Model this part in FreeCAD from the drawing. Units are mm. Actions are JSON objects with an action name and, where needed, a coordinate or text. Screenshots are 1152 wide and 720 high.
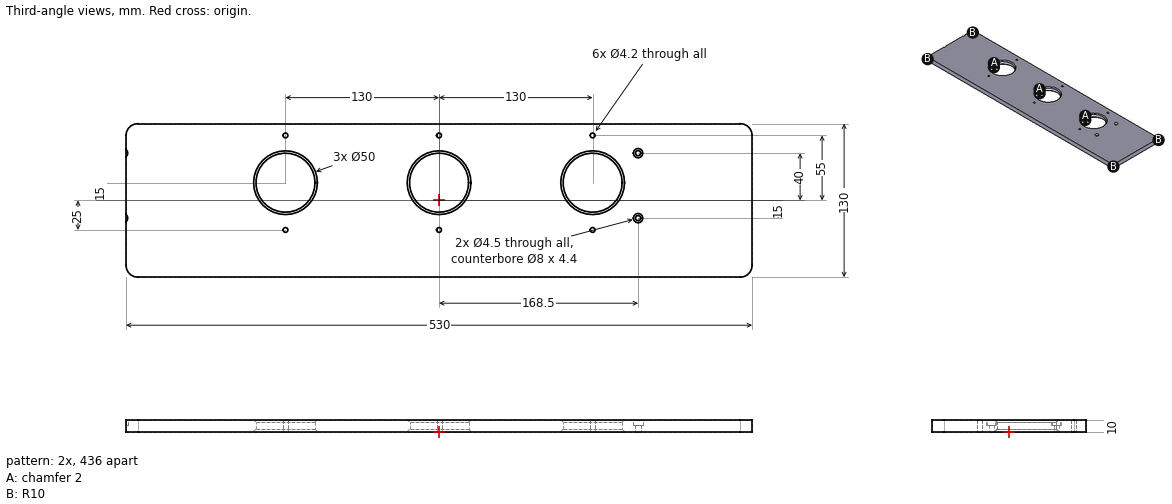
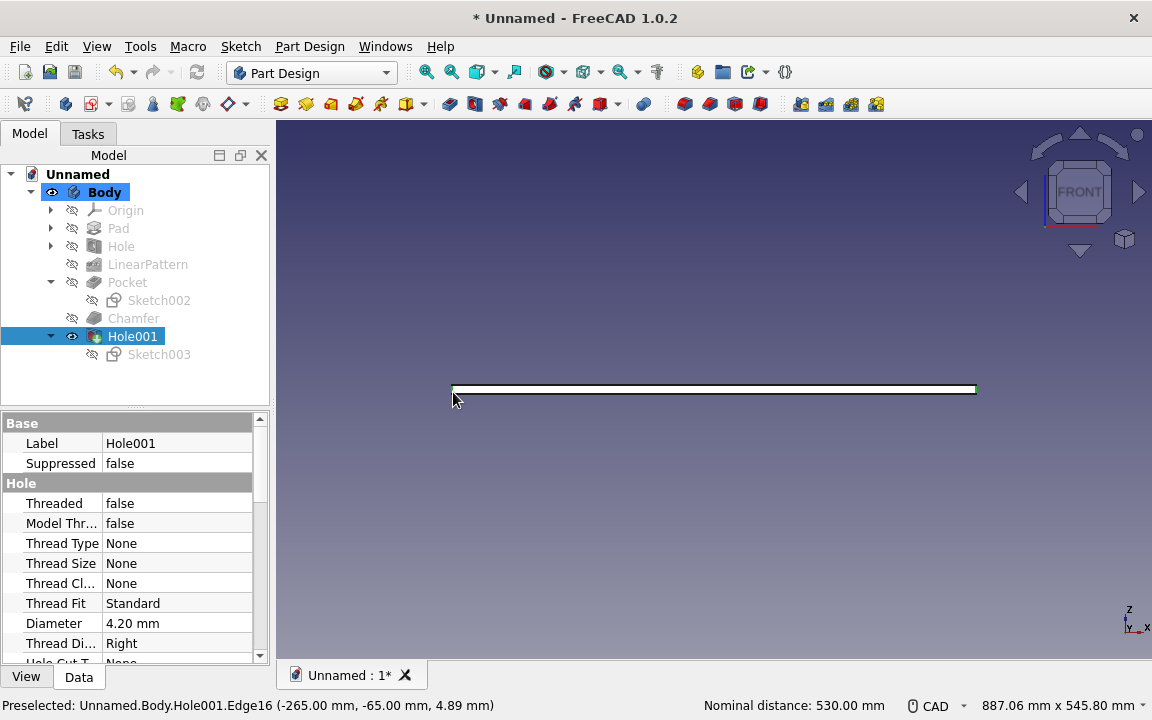
{"action": "key", "text": "3"}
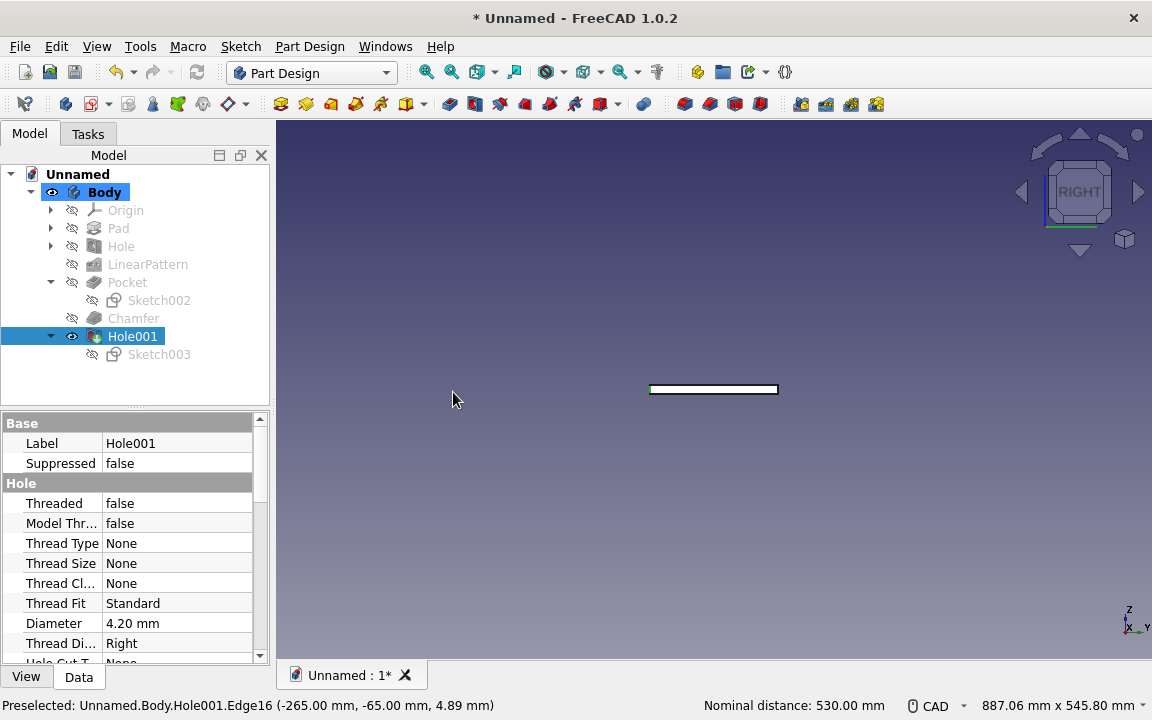
{"action": "left_click", "coordinate": [427, 72]}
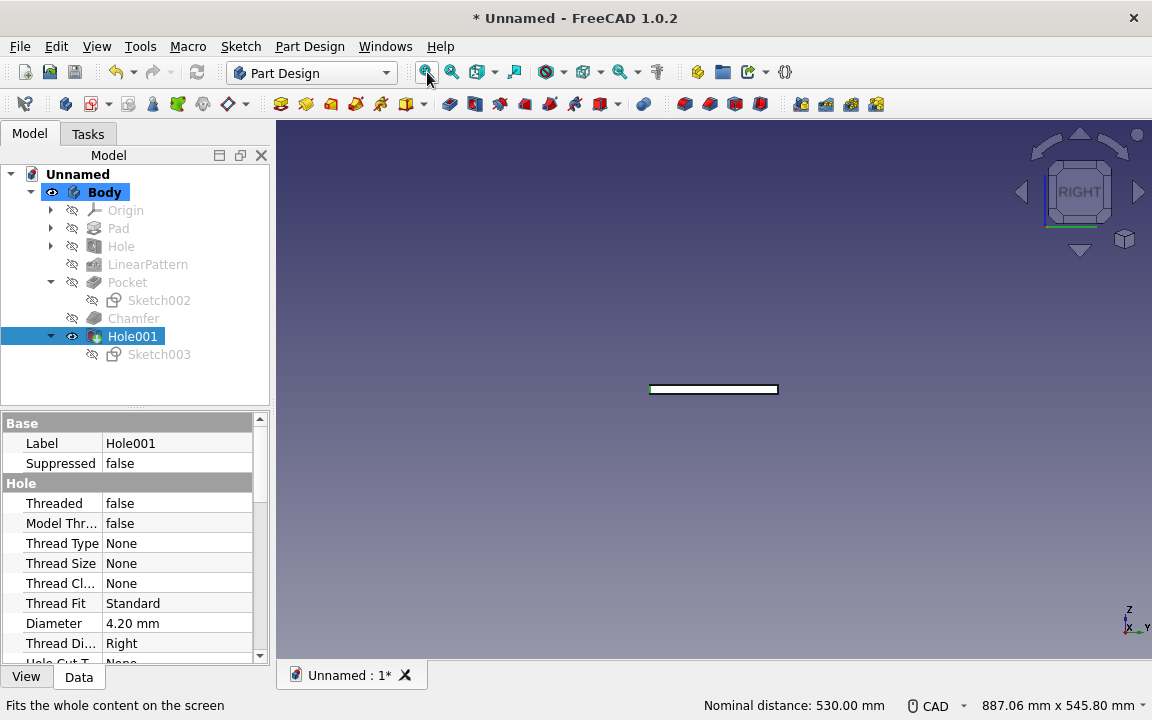
{"action": "scroll", "coordinate": [778, 388], "scroll_direction": "up", "scroll_amount": 7}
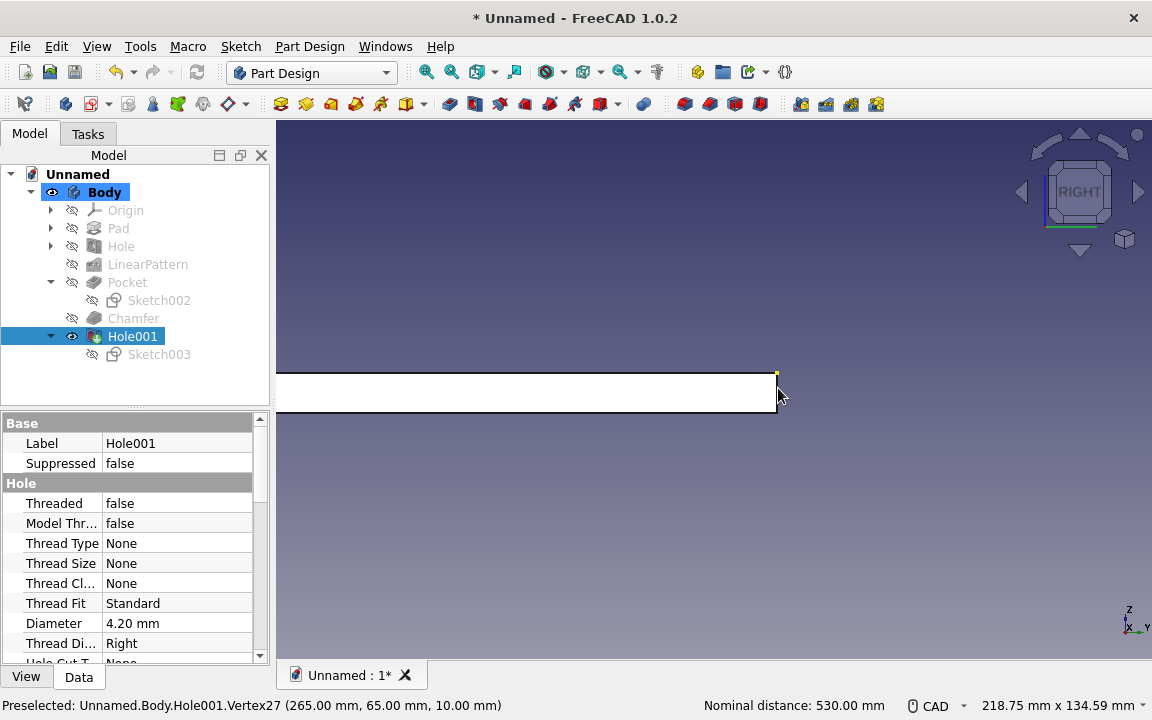
{"action": "left_click", "coordinate": [777, 392], "text": "ctrl"}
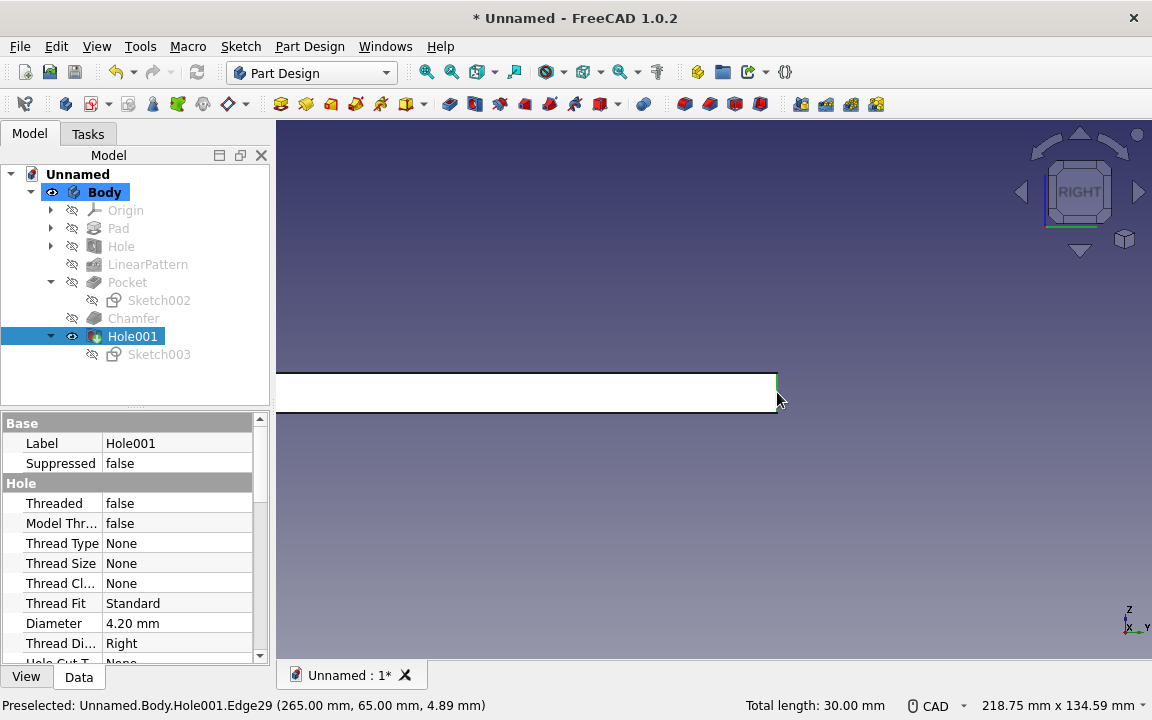
{"action": "left_click", "coordinate": [427, 72]}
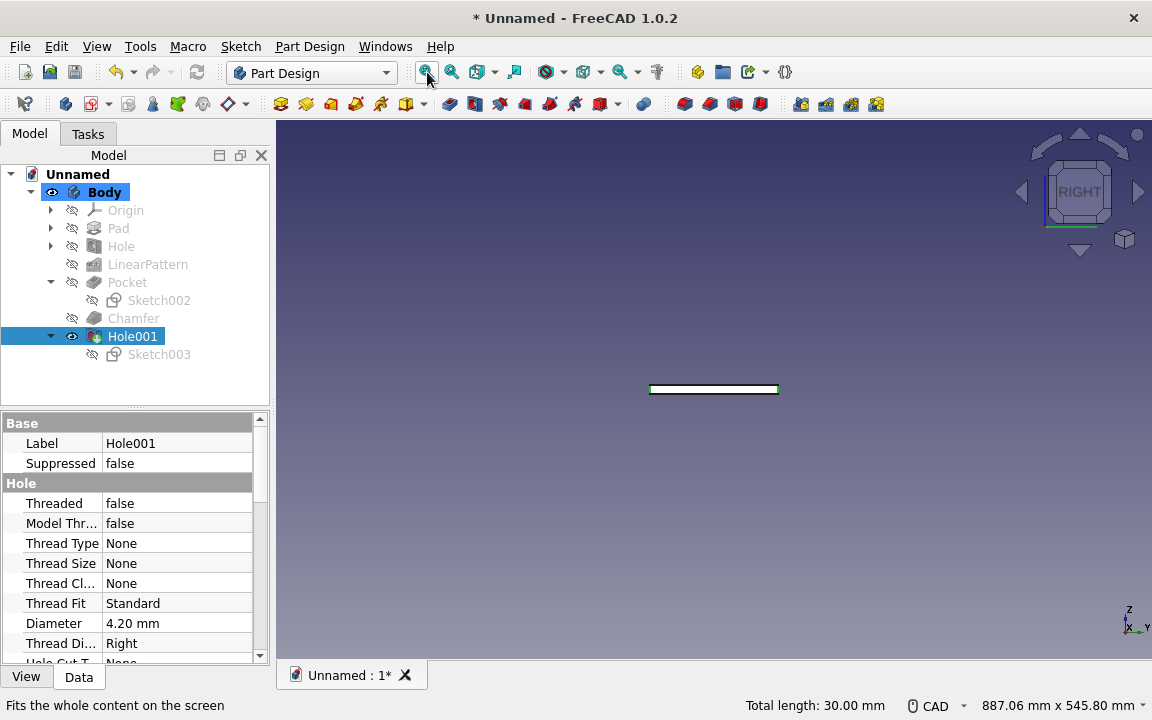
{"action": "key", "text": "5"}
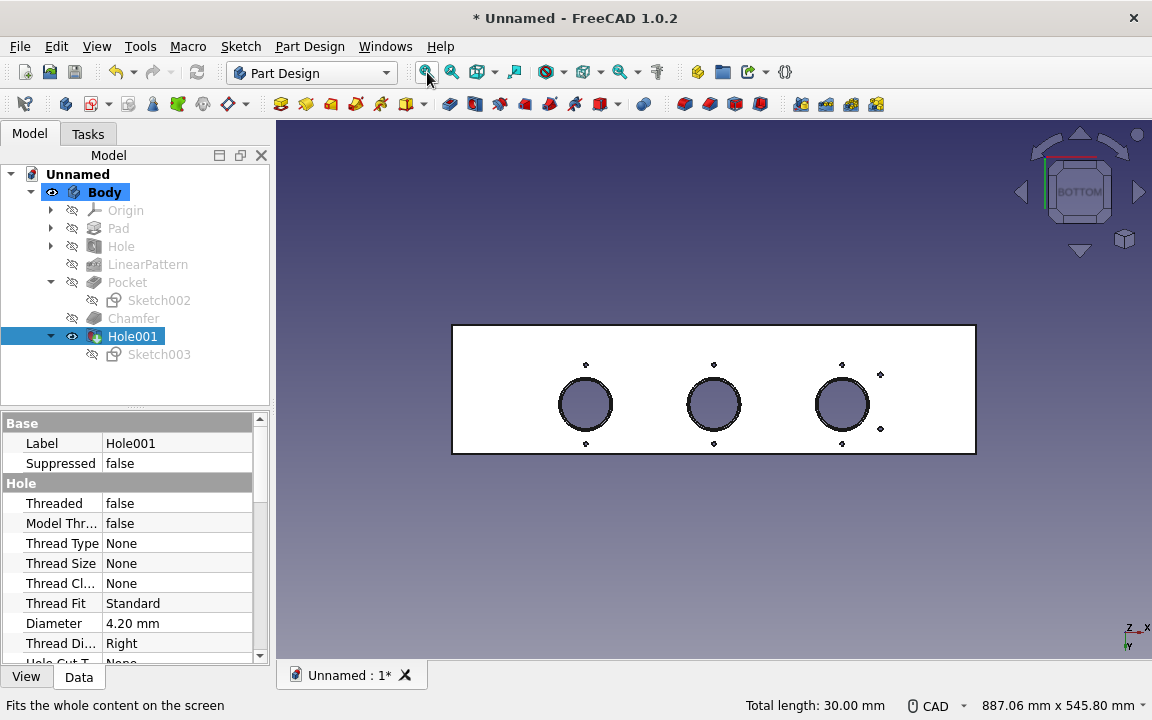
{"action": "scroll", "coordinate": [452, 453], "scroll_direction": "up", "scroll_amount": 7}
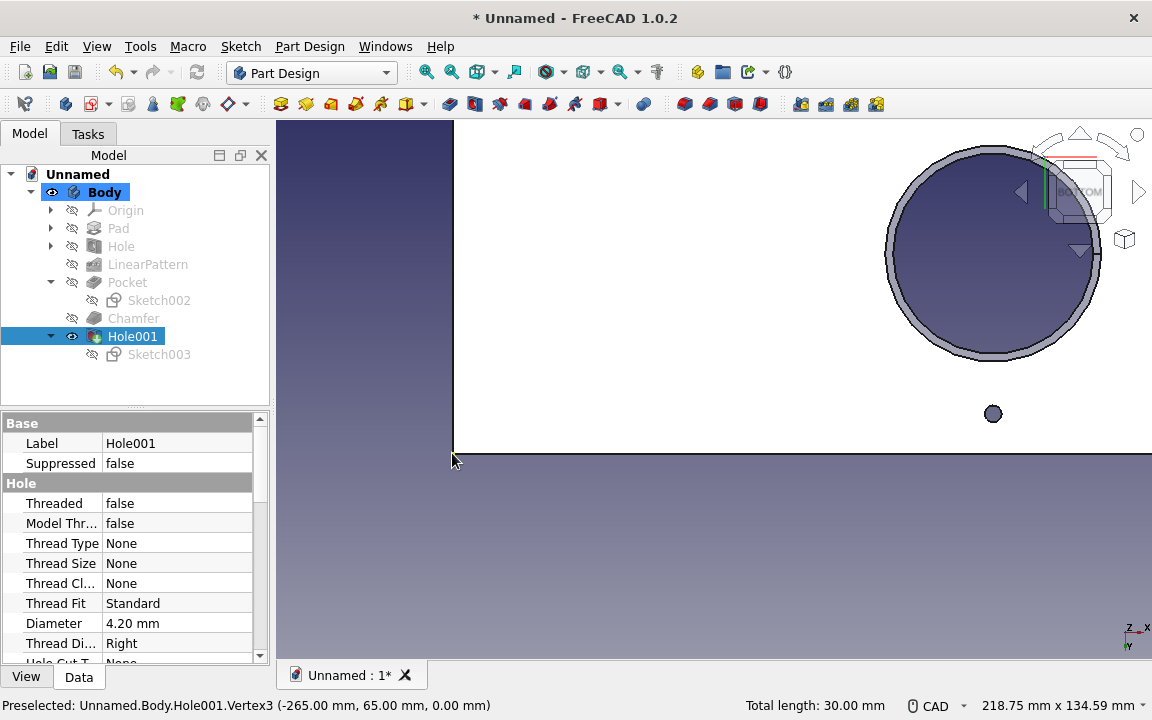
{"action": "left_click", "coordinate": [427, 72]}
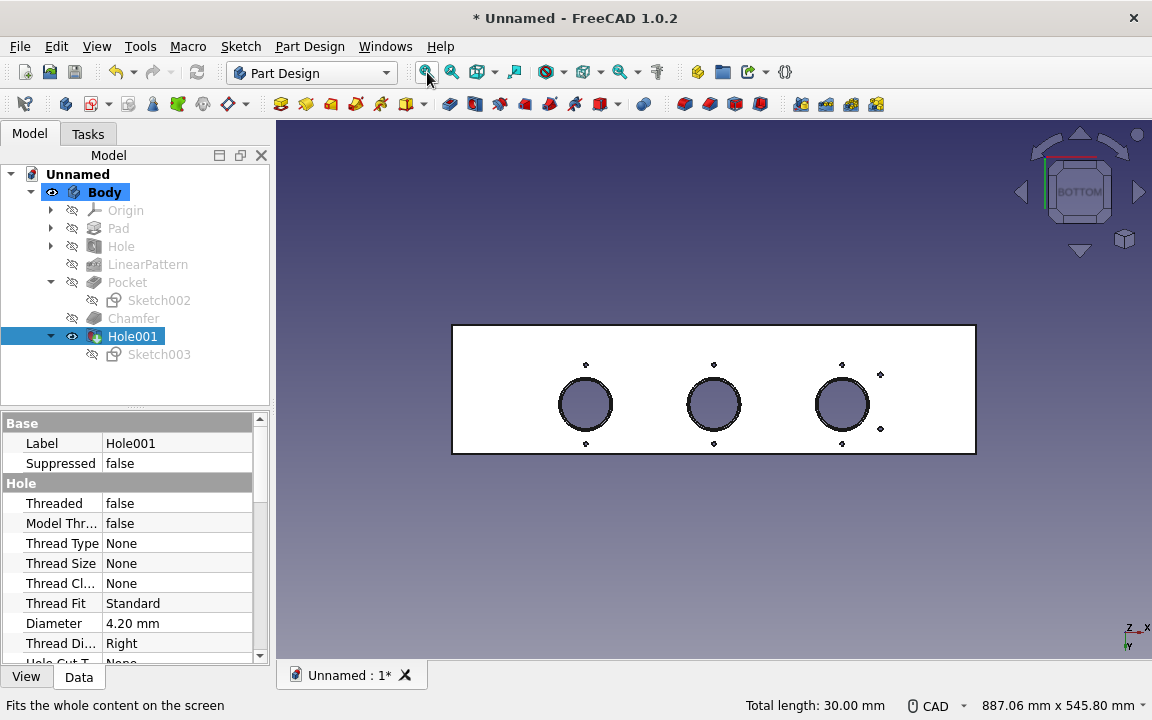
{"action": "key", "text": "4"}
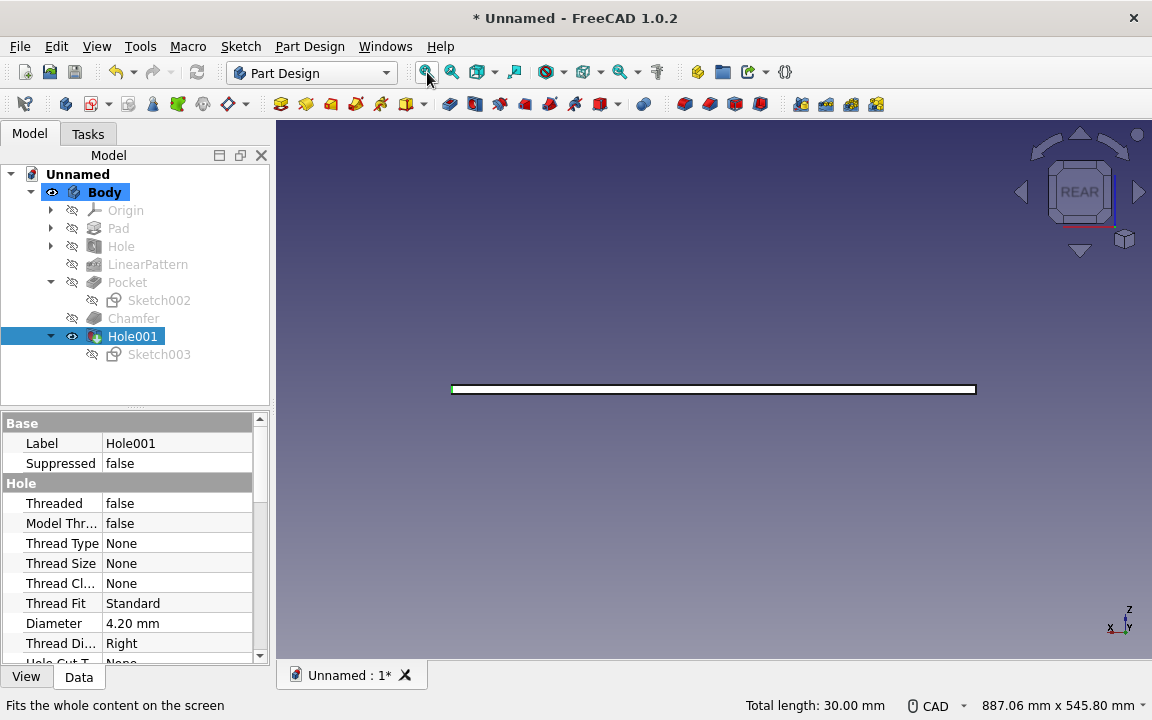
{"action": "scroll", "coordinate": [976, 388], "scroll_direction": "up", "scroll_amount": 7}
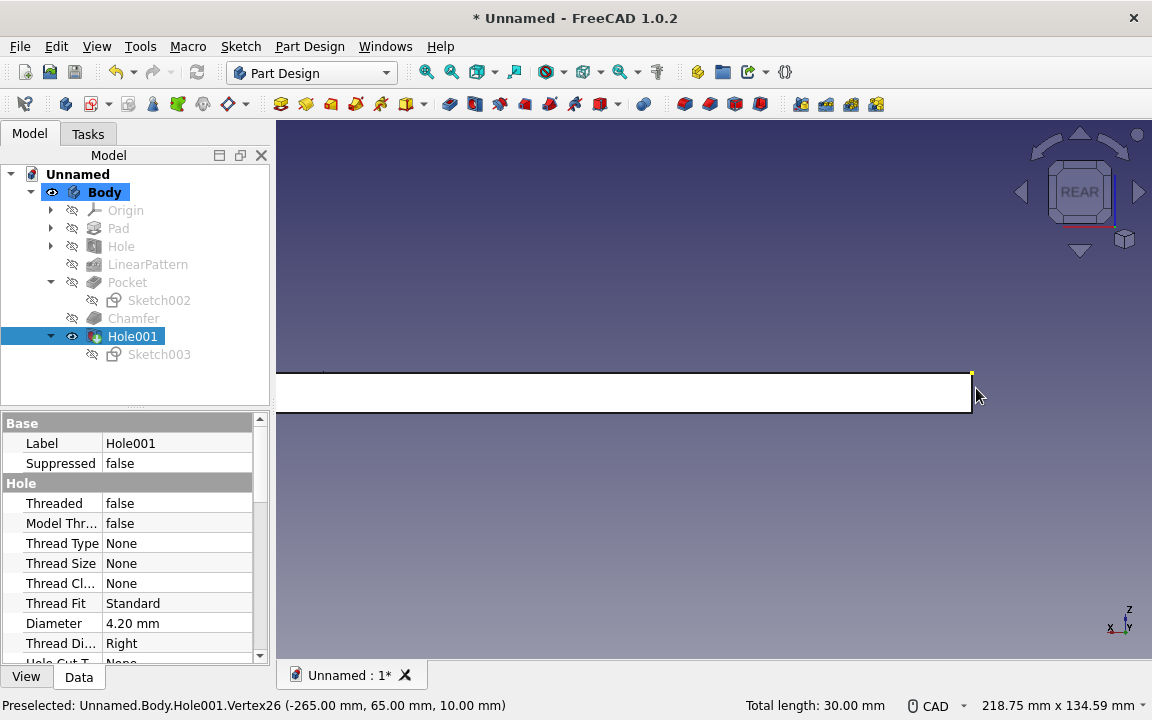
{"action": "left_click", "coordinate": [972, 392], "text": "ctrl"}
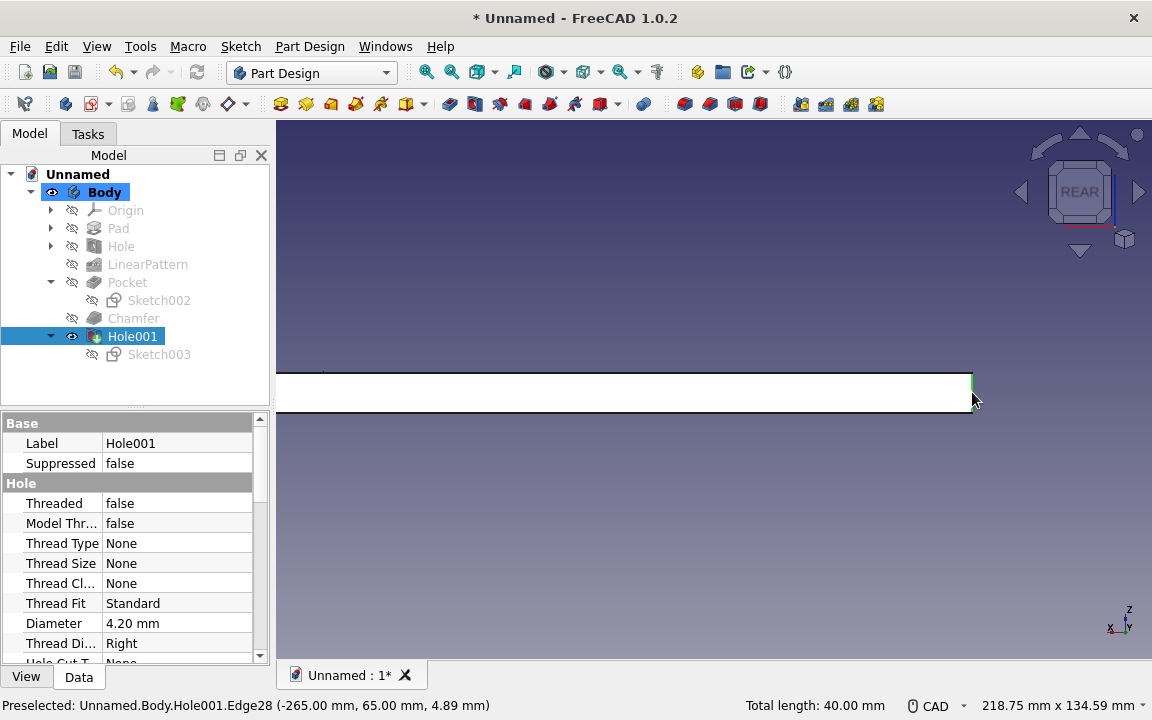
{"action": "left_click", "coordinate": [685, 104]}